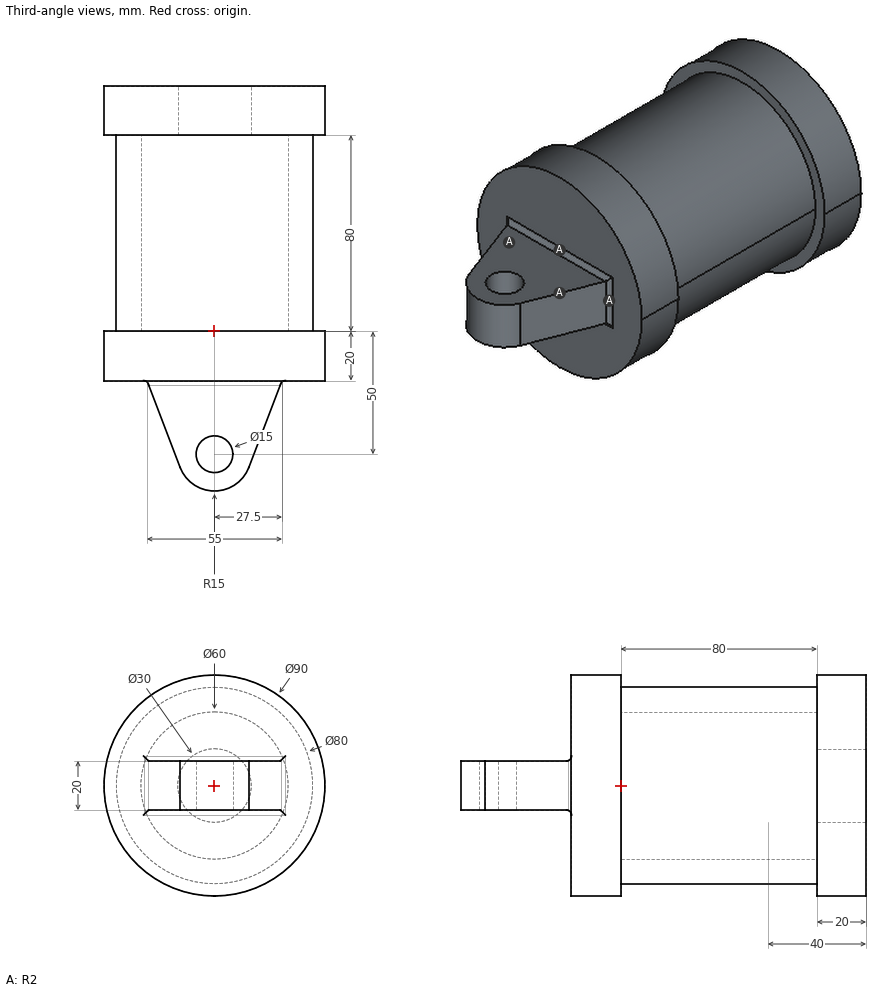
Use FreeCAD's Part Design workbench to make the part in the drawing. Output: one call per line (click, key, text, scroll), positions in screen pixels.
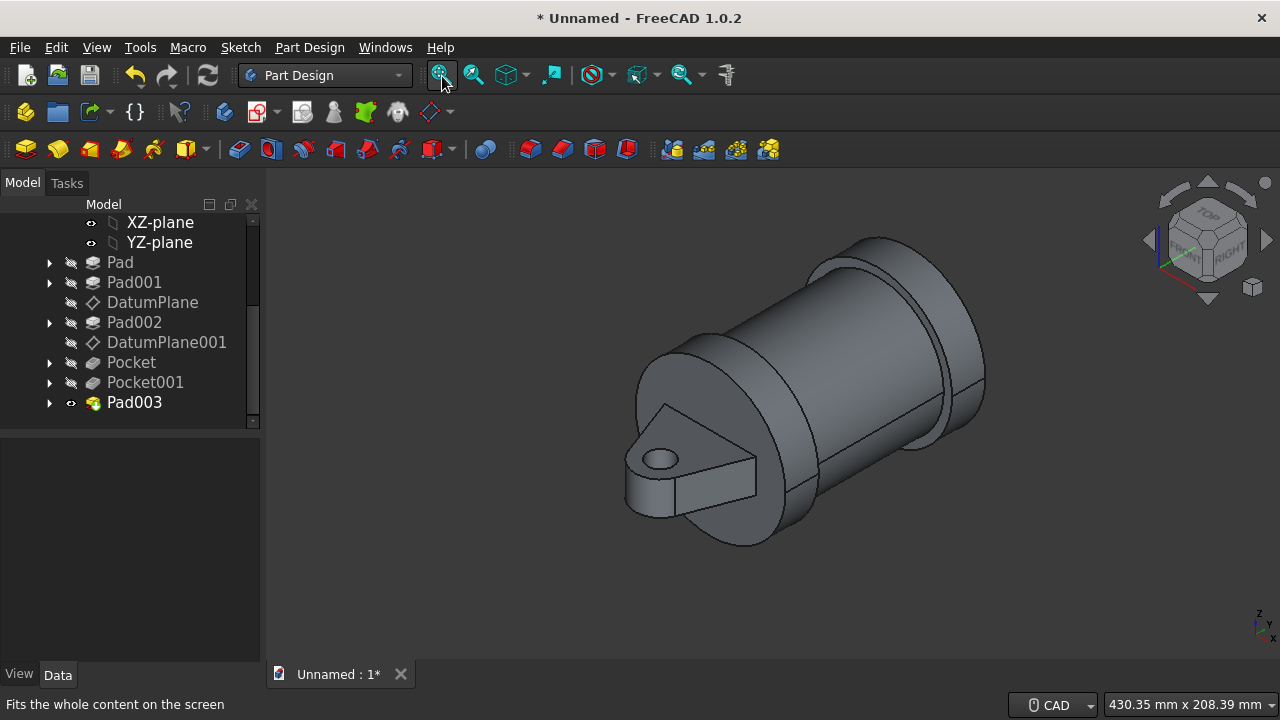
key(2)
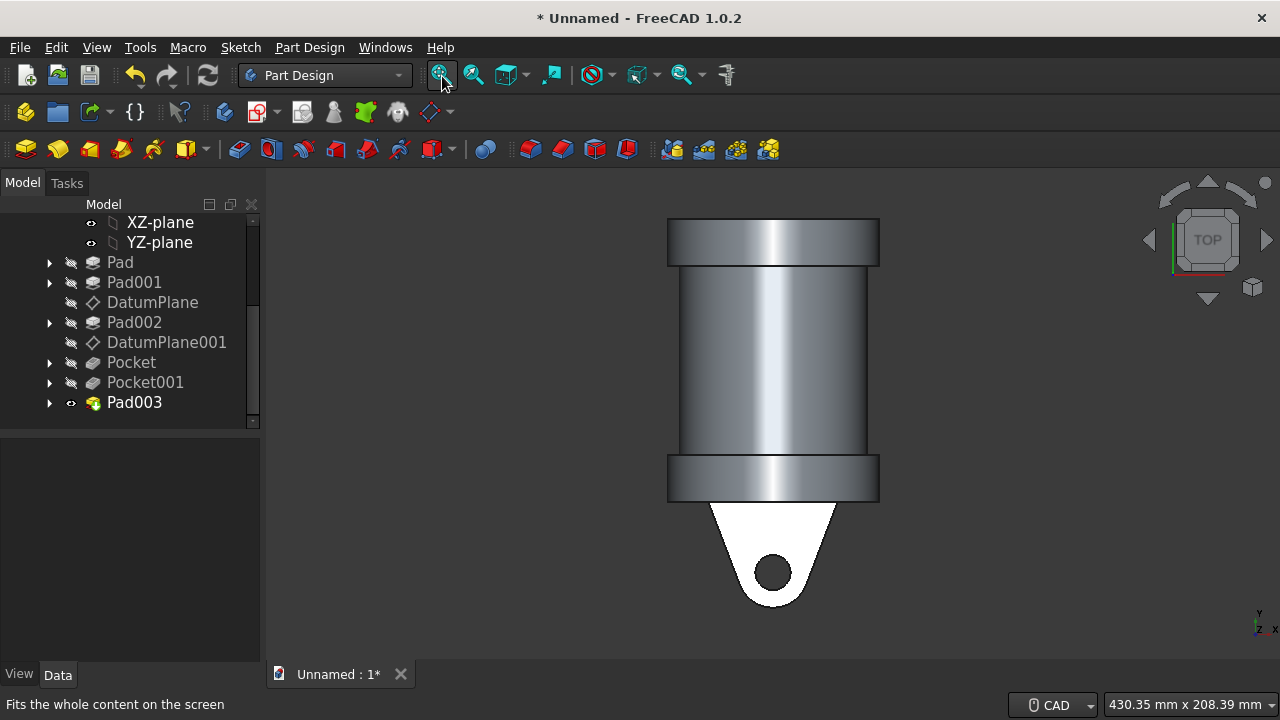
key(1)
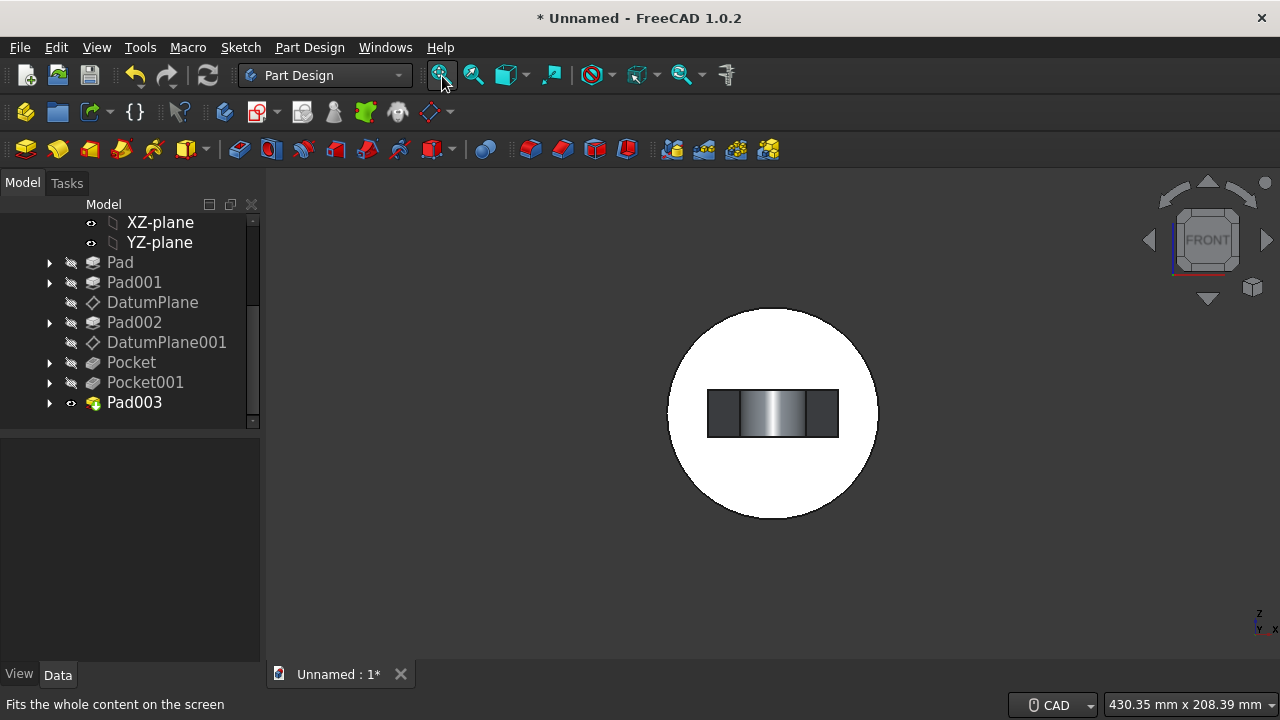
key(v)
key(f)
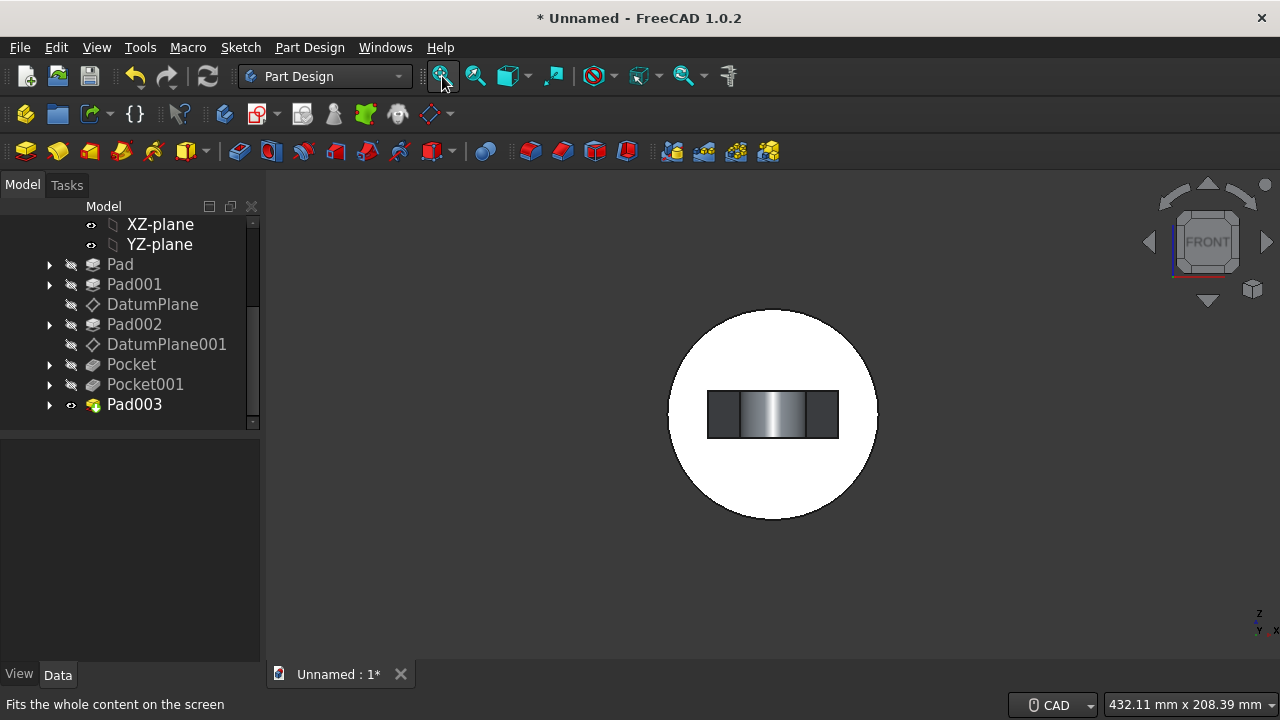
key(3)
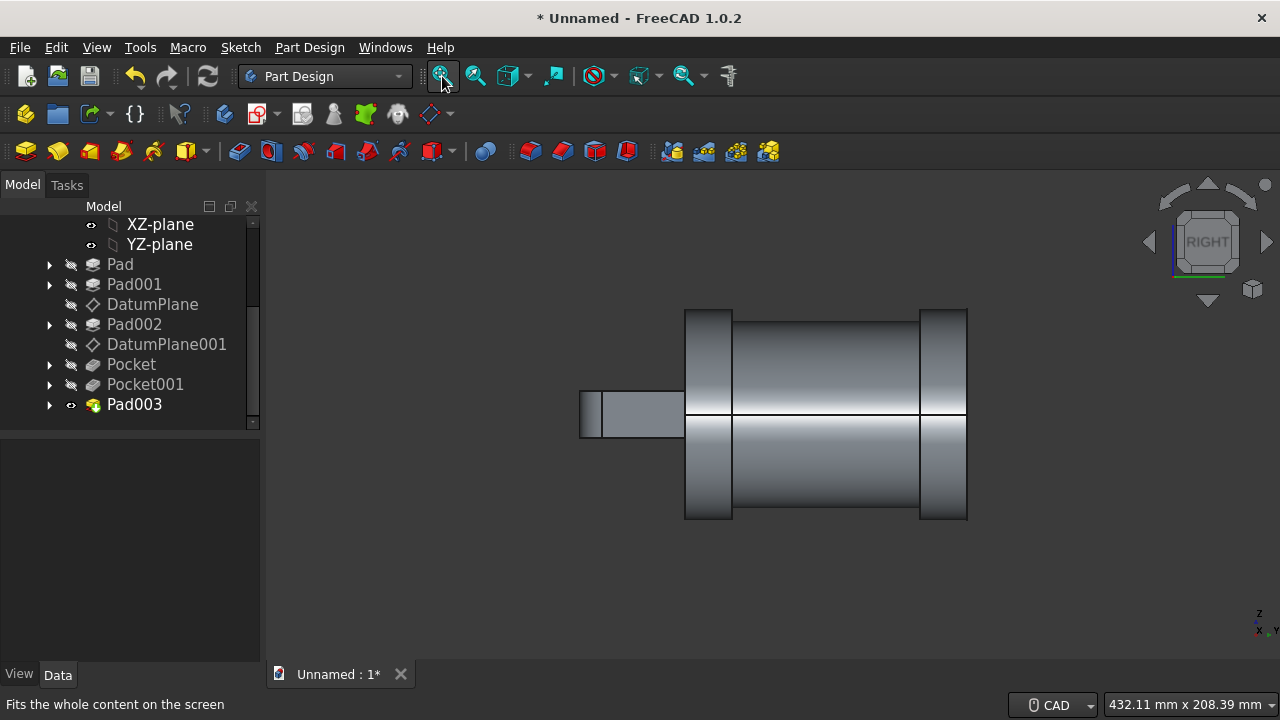
key(v)
key(f)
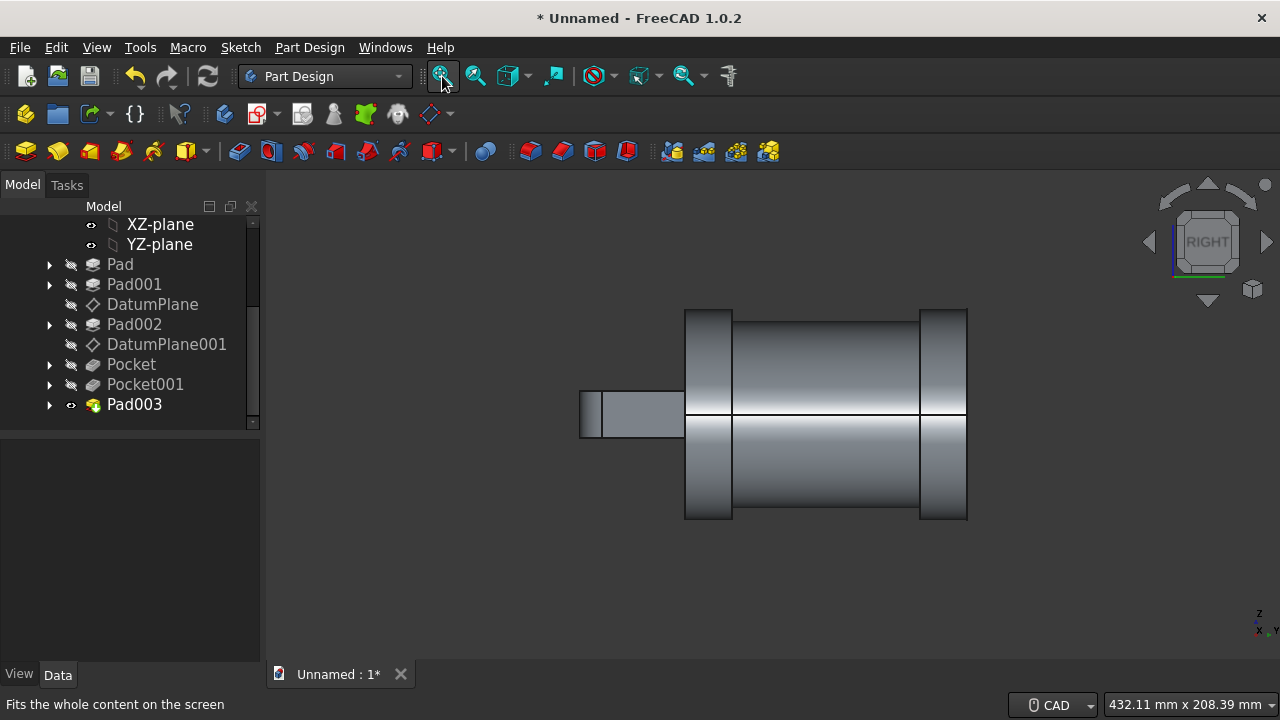
key(5)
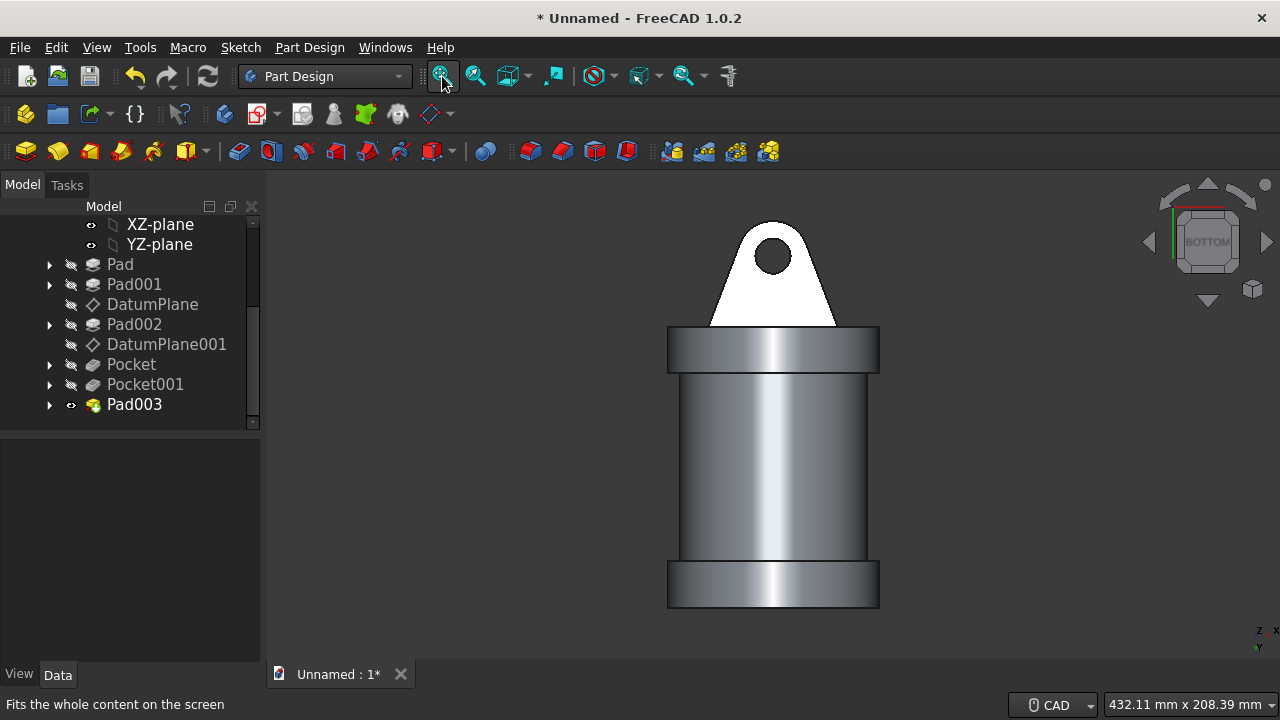
key(4)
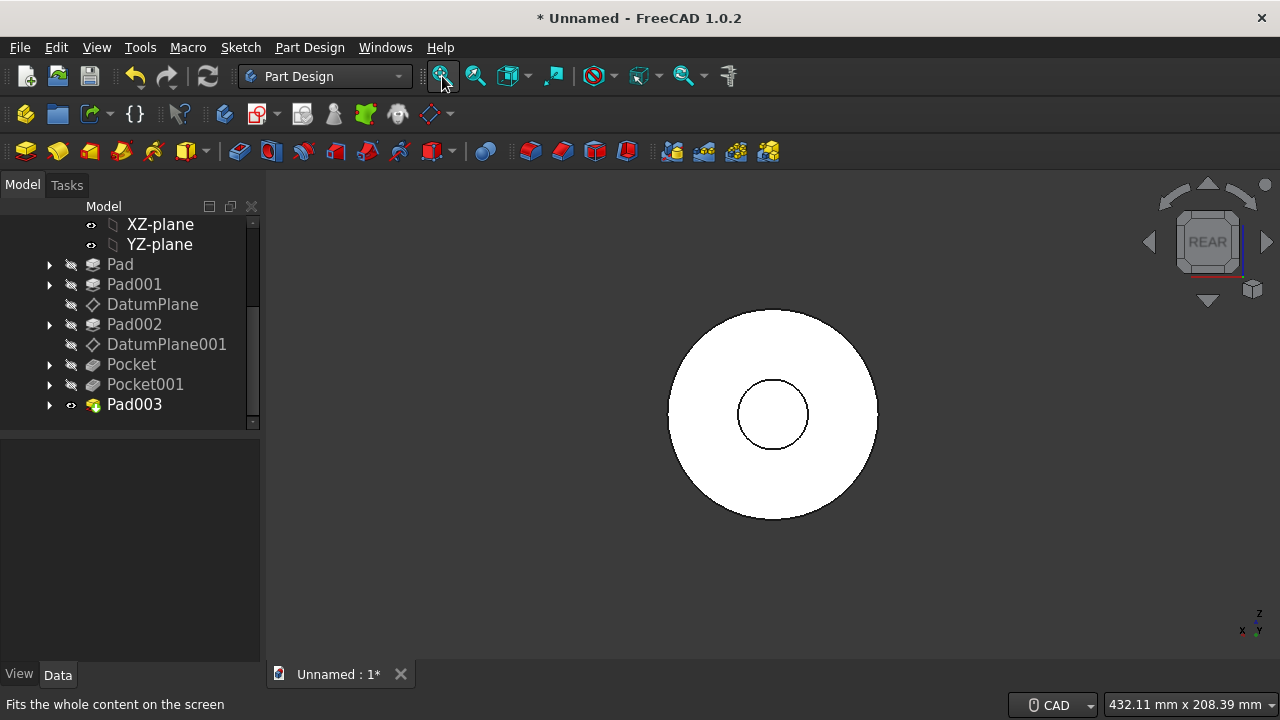
click(444, 76)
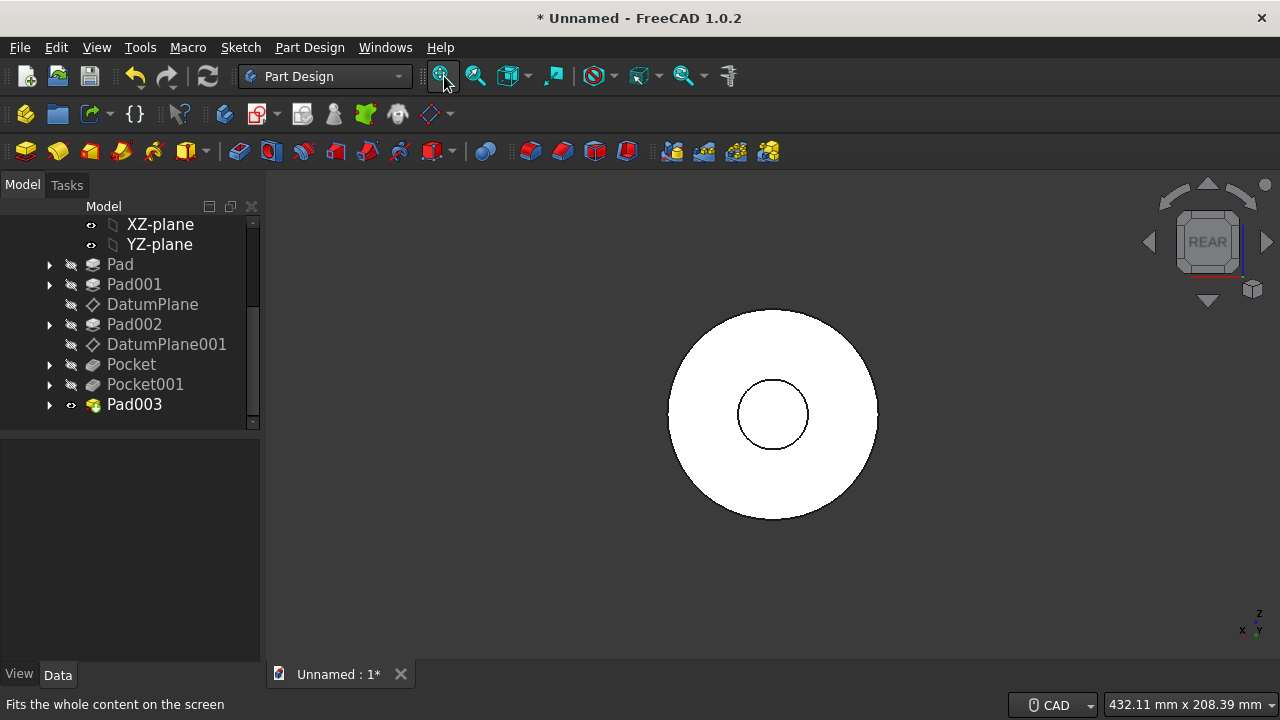
key(6)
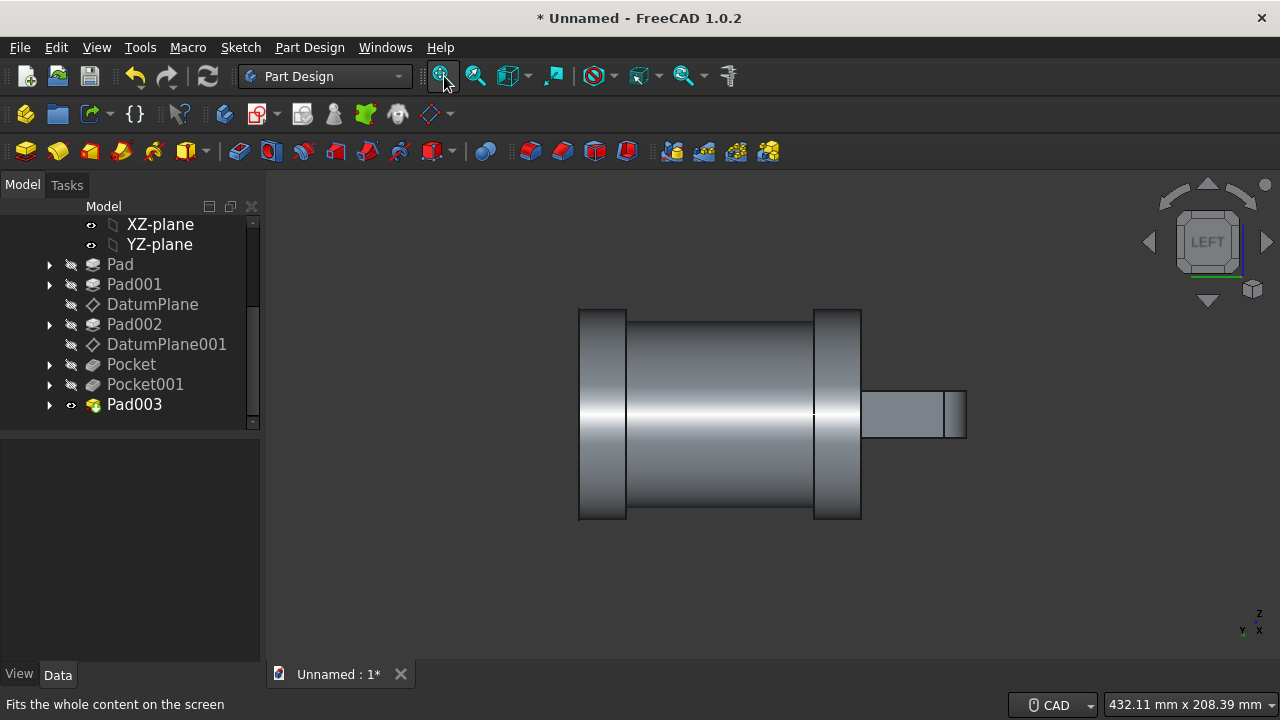
key(v)
key(f)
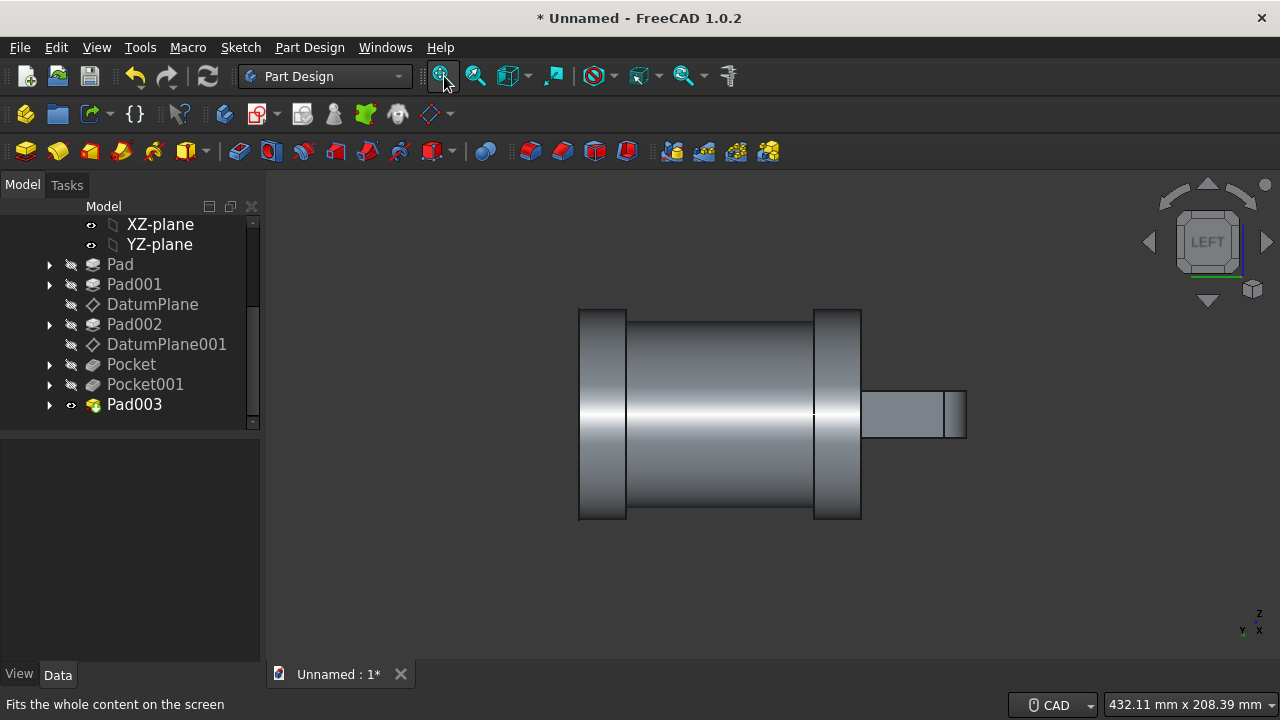
key(v)
key(3)